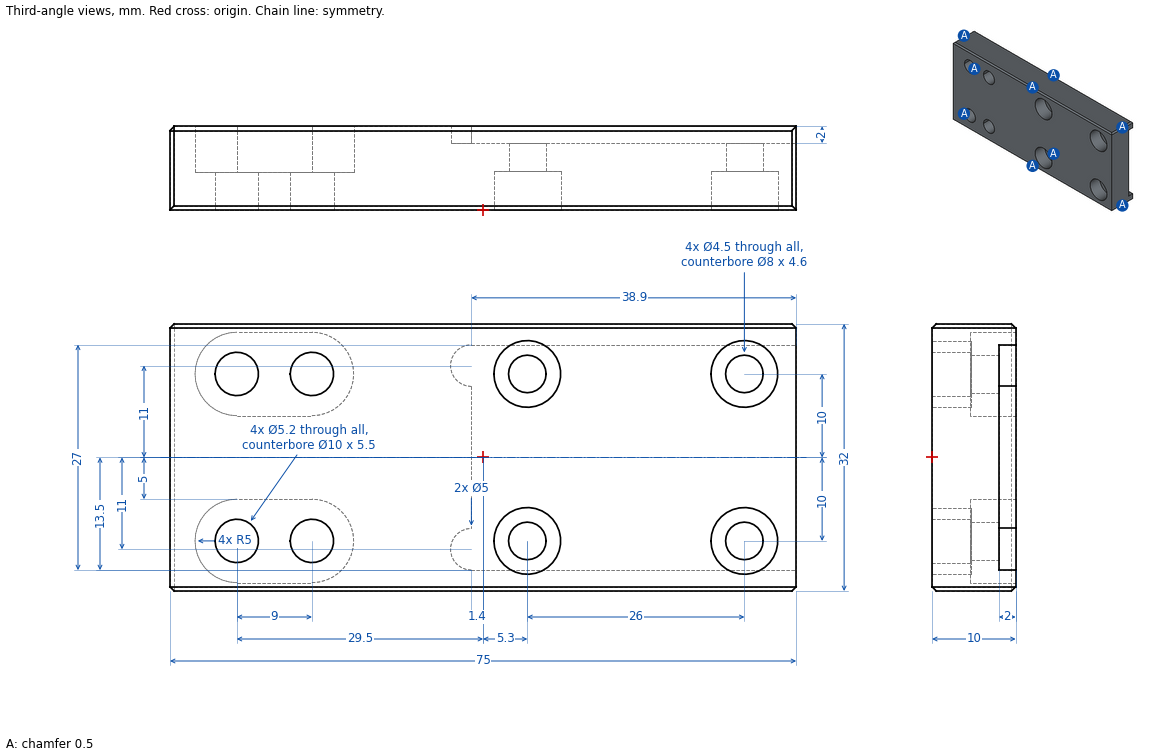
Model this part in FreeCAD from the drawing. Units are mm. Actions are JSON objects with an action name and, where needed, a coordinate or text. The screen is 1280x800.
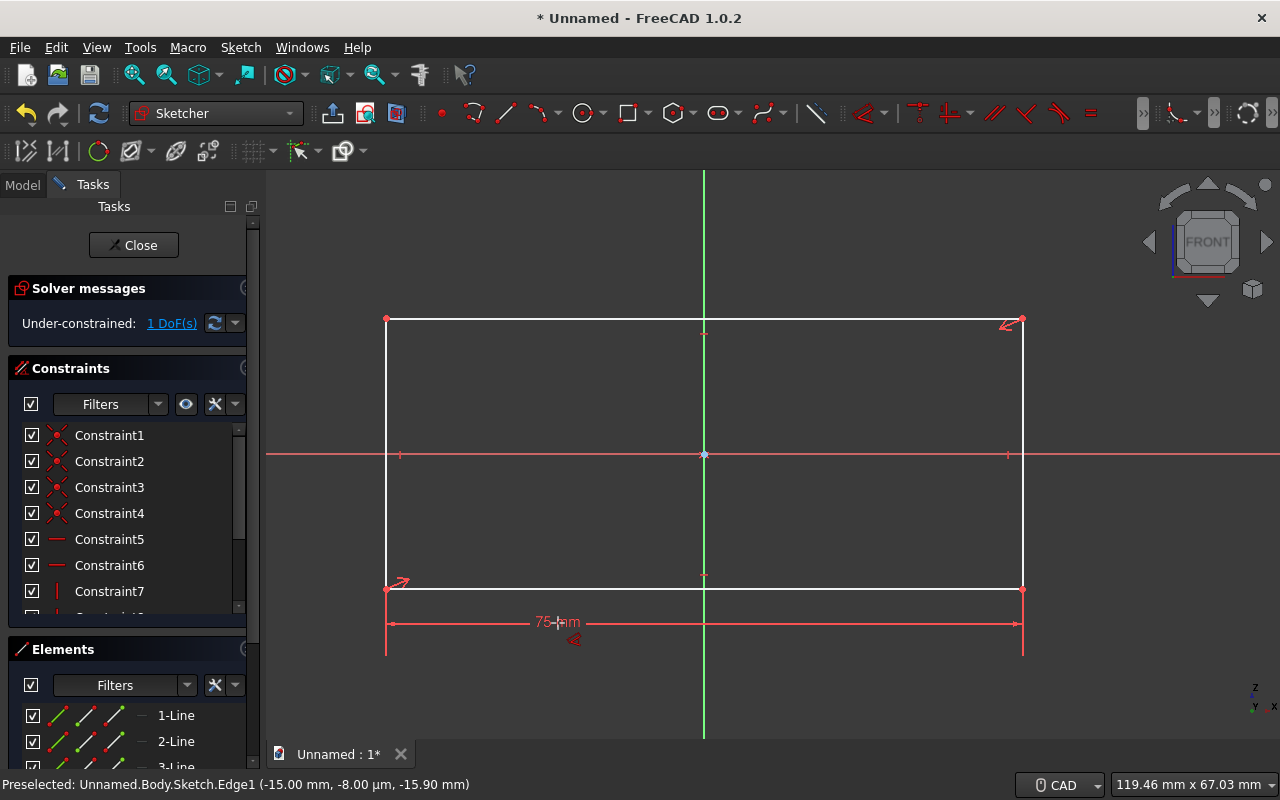
{"action": "left_click", "coordinate": [1023, 508]}
{"action": "left_click", "coordinate": [1057, 392]}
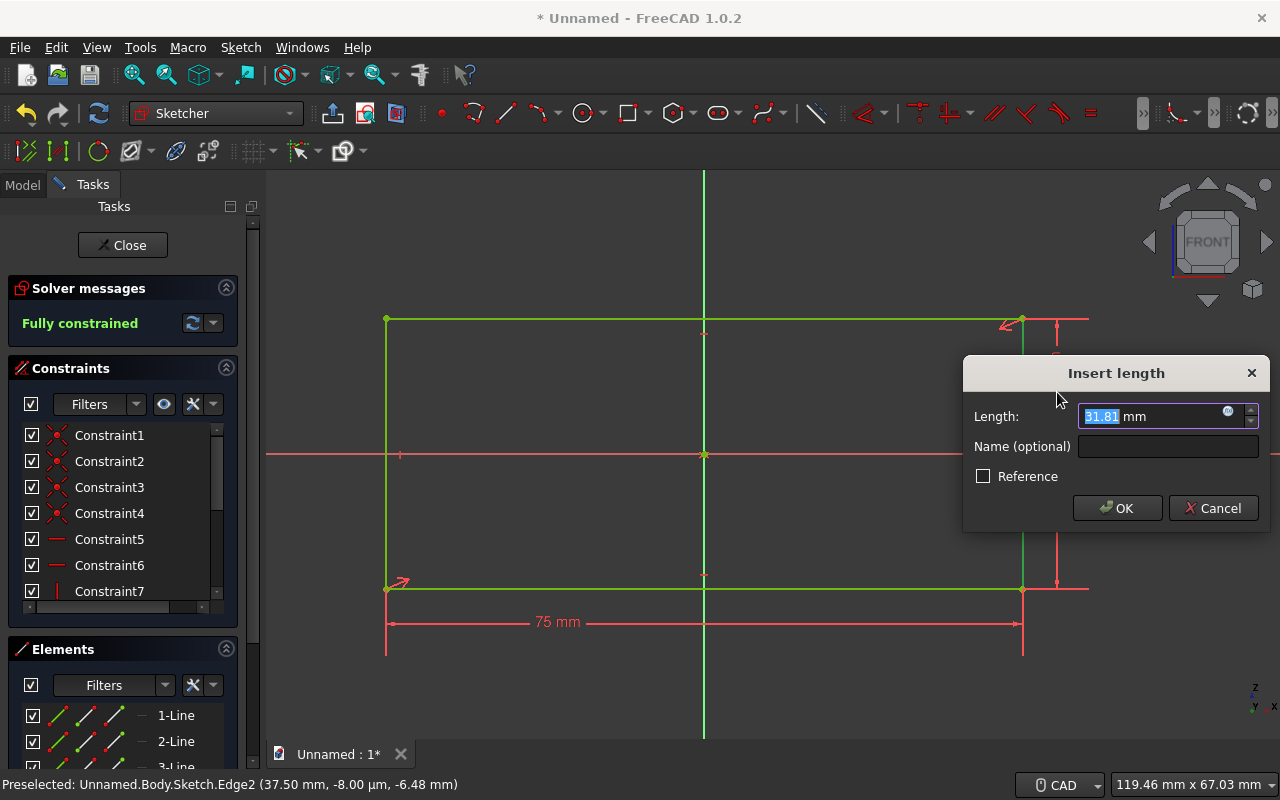
{"action": "type", "text": "32"}
{"action": "key", "text": "Return"}
{"action": "key", "text": "Escape"}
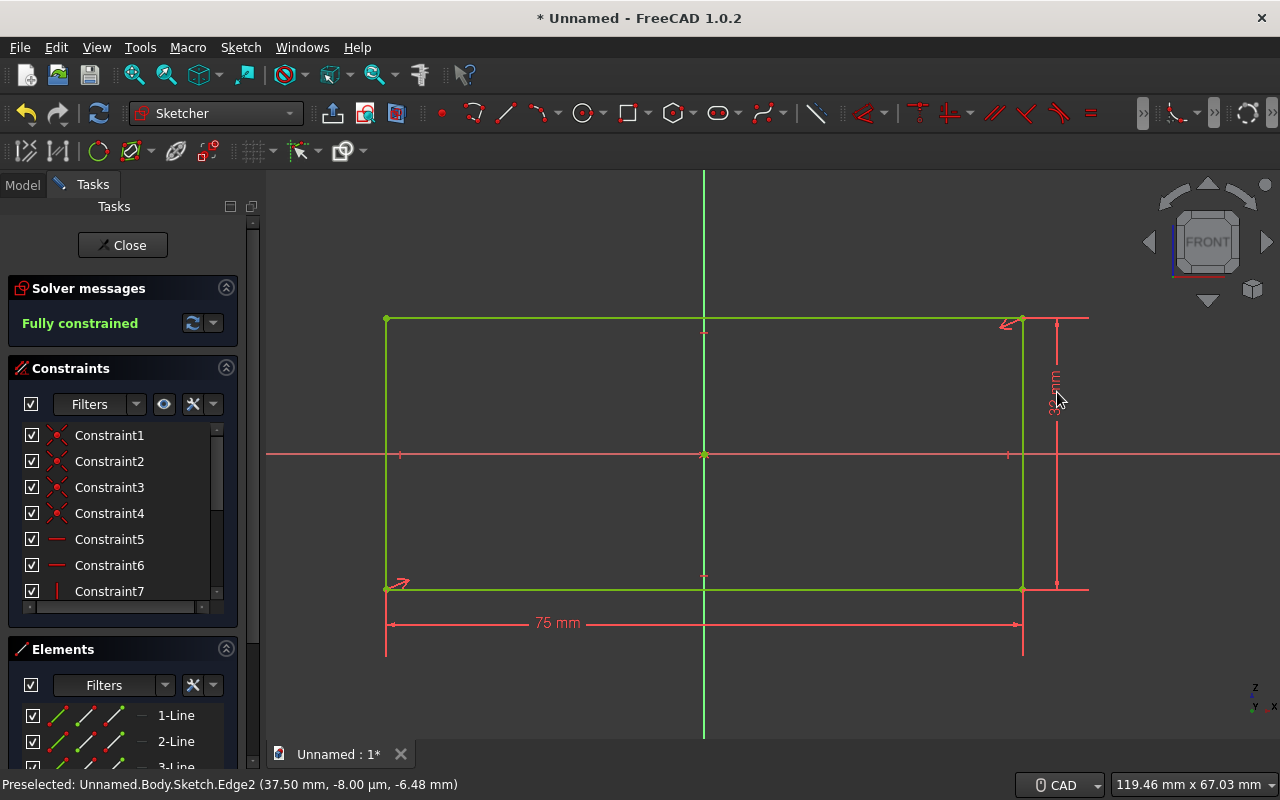
{"action": "left_click", "coordinate": [123, 245]}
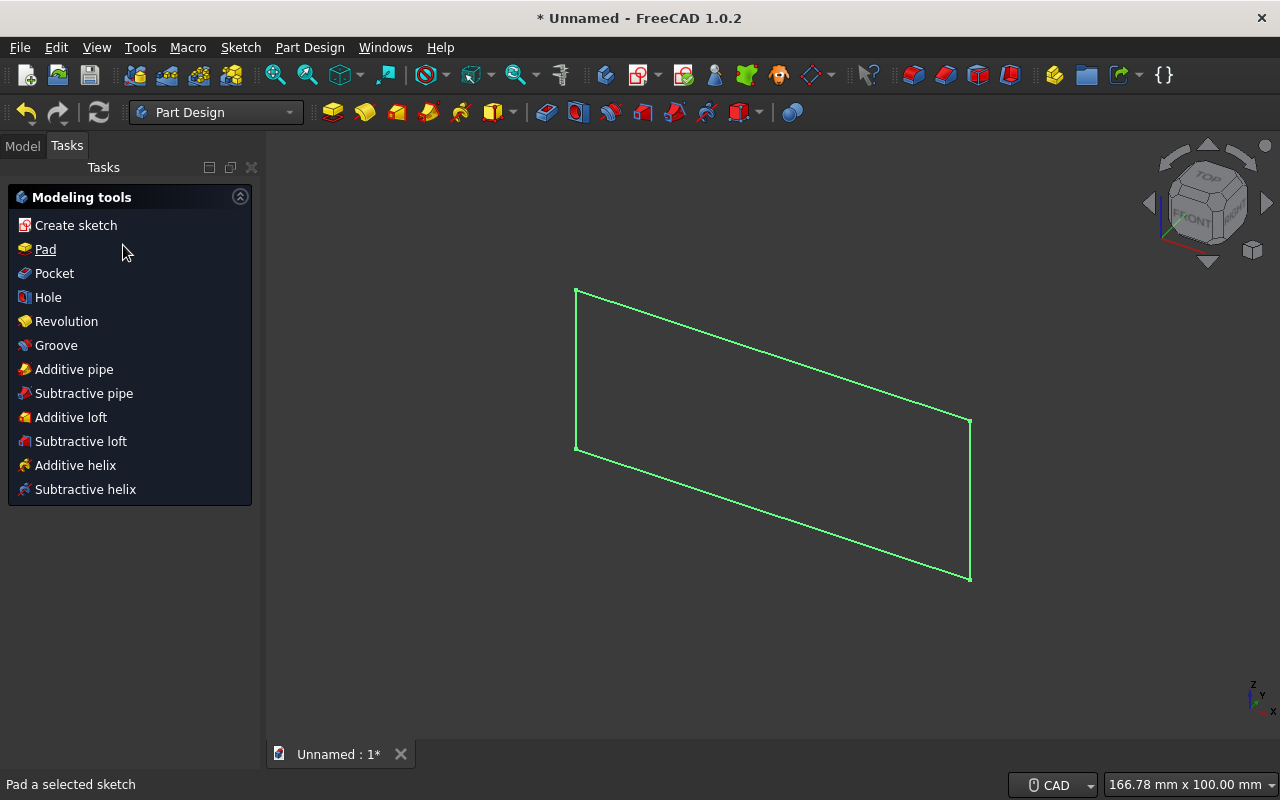
{"action": "left_click", "coordinate": [334, 112]}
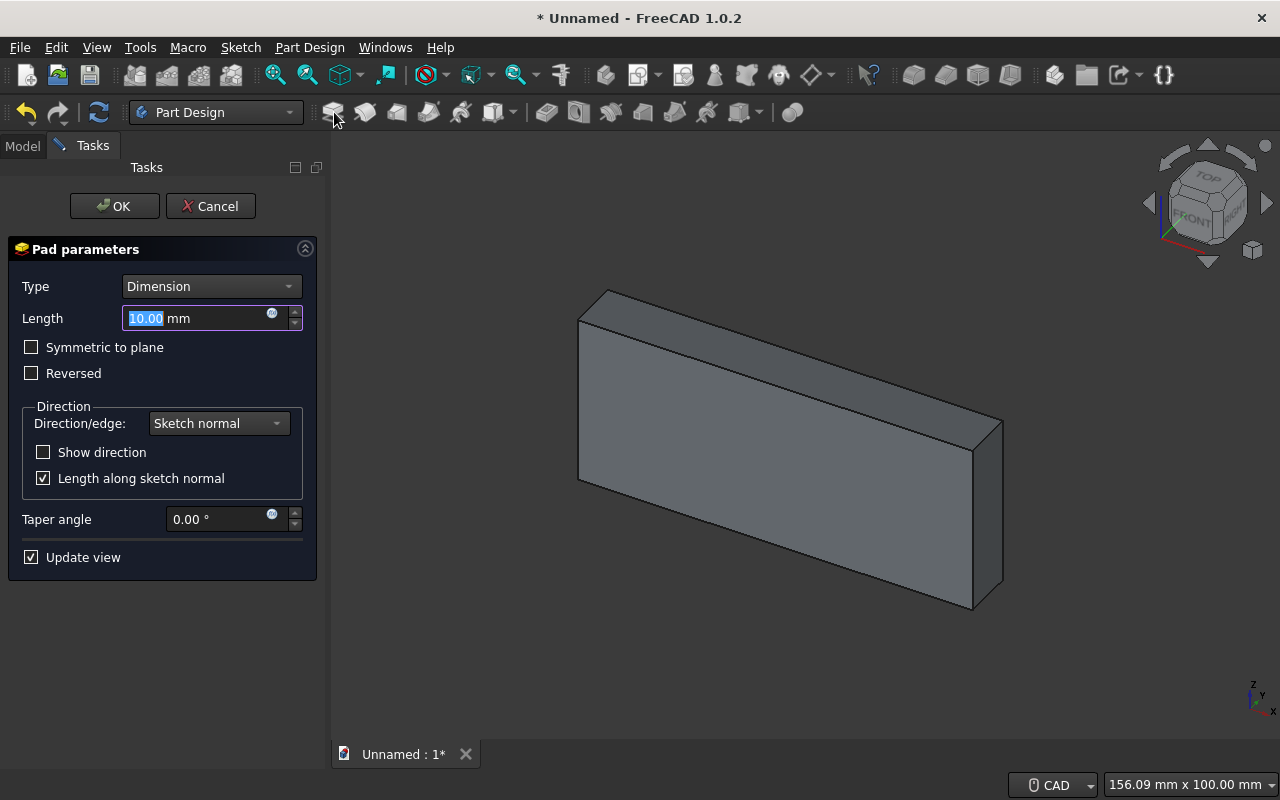
{"action": "type", "text": "10"}
{"action": "key", "text": "Tab"}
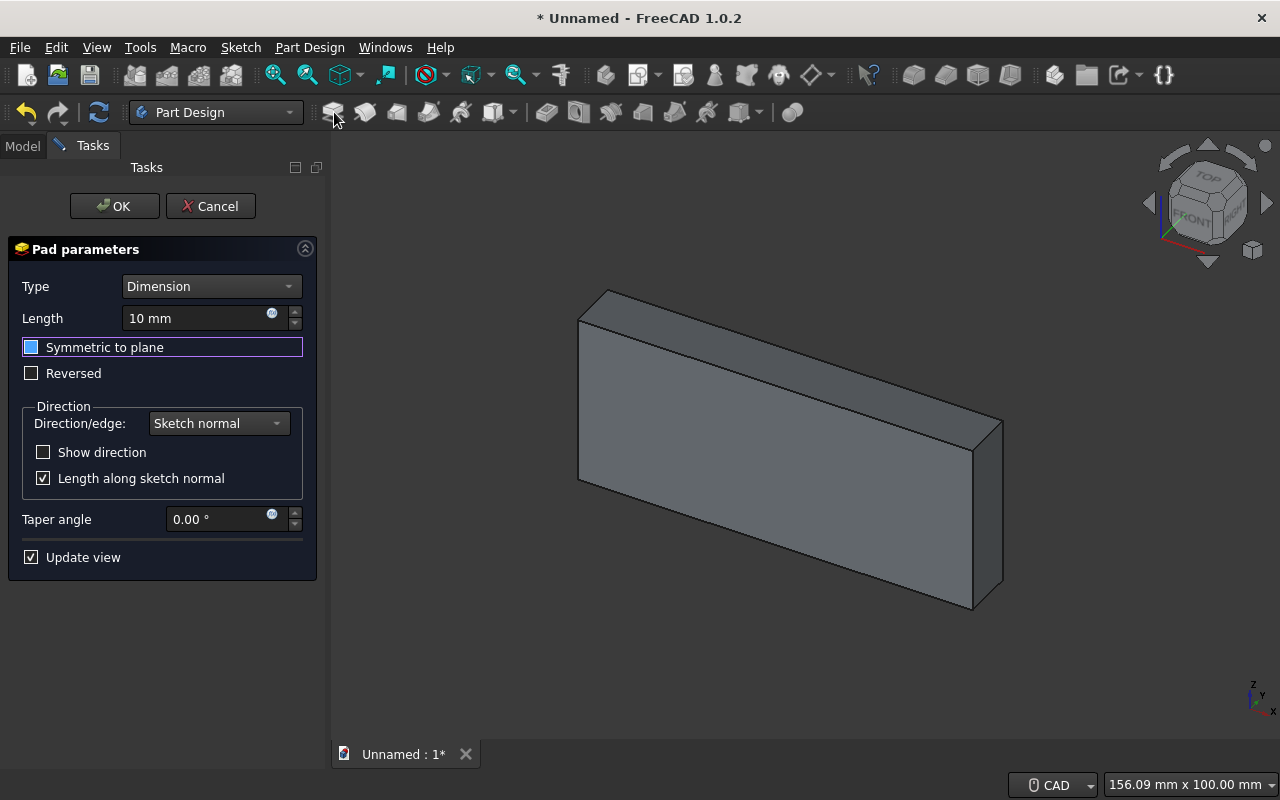
{"action": "left_click", "coordinate": [30, 373]}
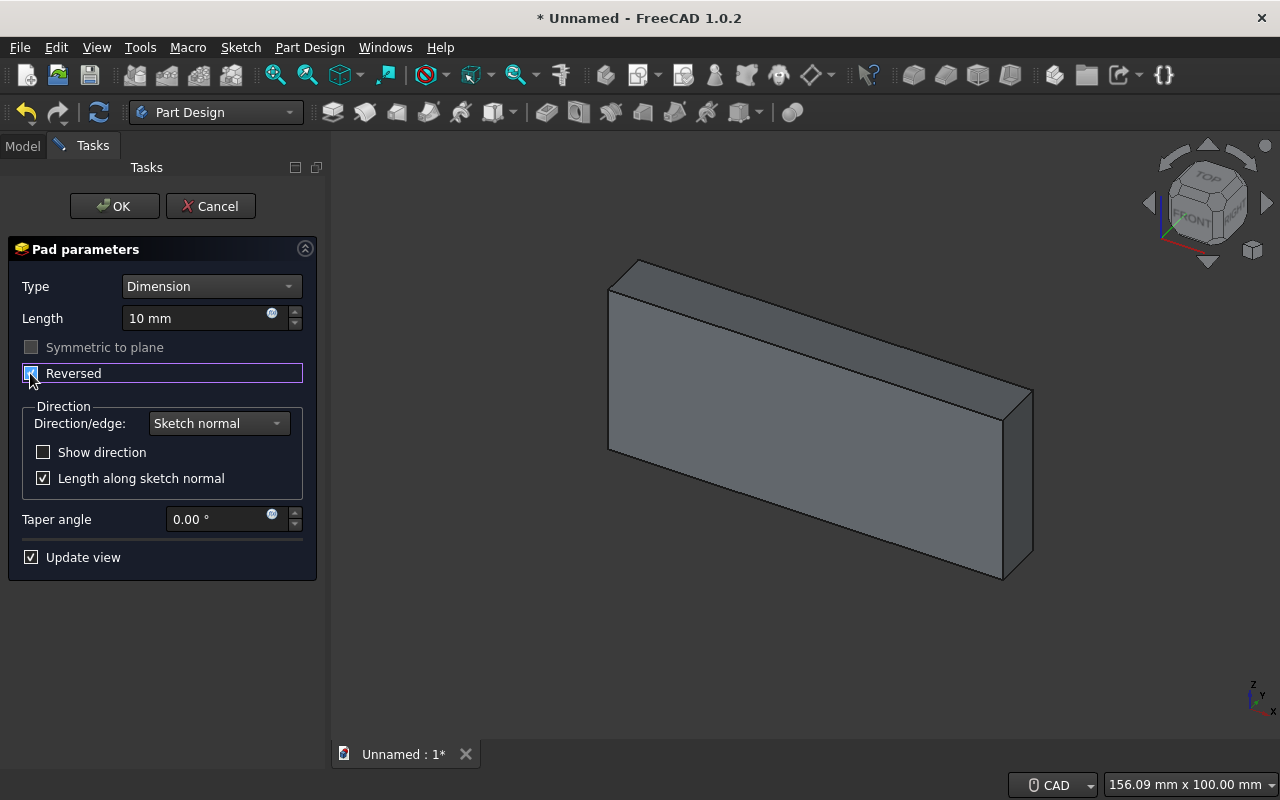
{"action": "left_click", "coordinate": [115, 206]}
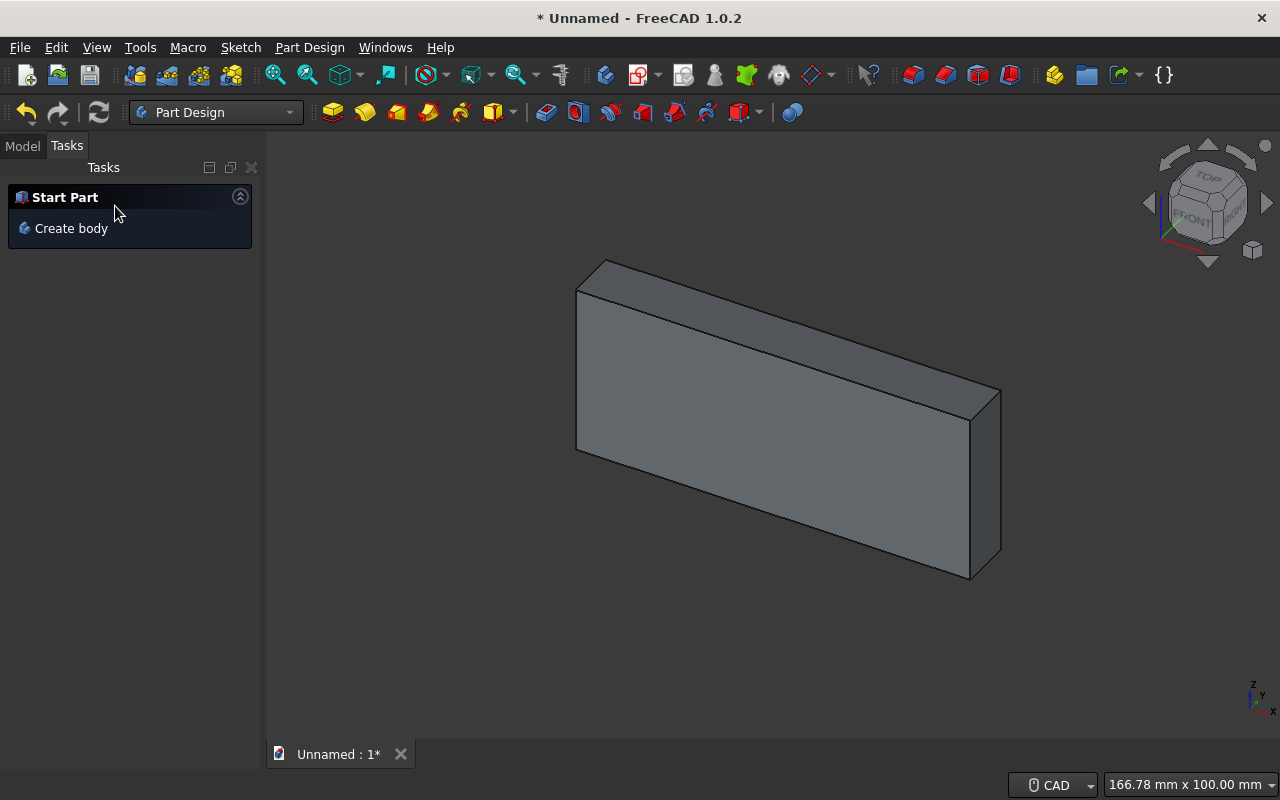
{"action": "key", "text": "4"}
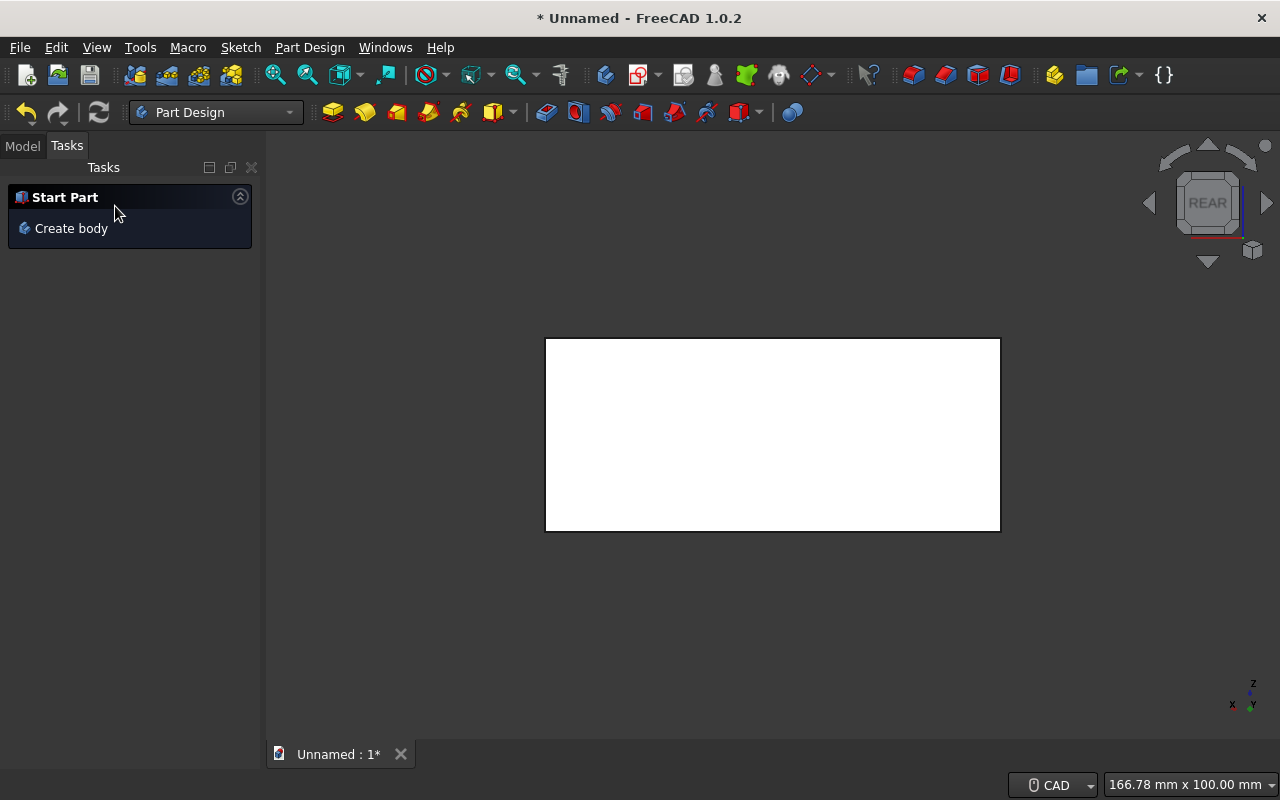
{"action": "left_click", "coordinate": [276, 76]}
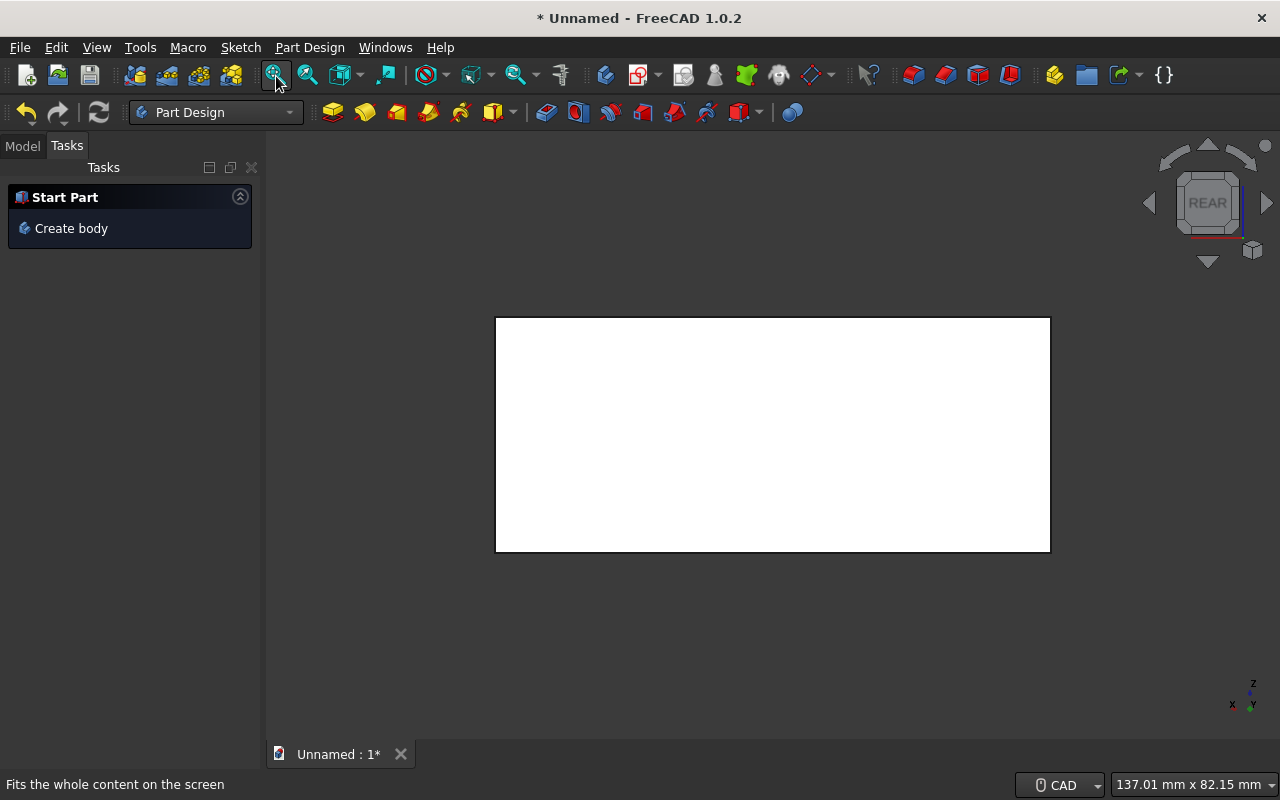
{"action": "left_click", "coordinate": [614, 434]}